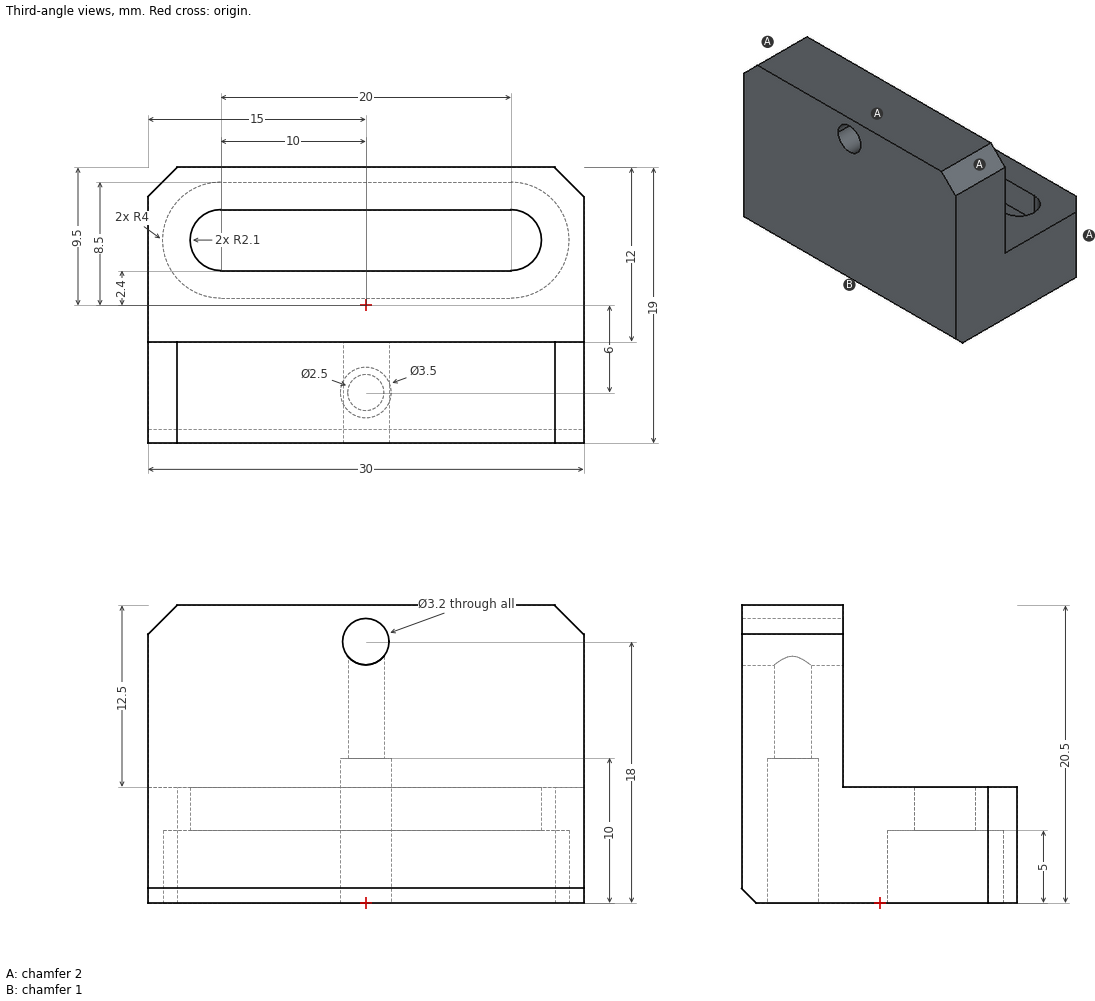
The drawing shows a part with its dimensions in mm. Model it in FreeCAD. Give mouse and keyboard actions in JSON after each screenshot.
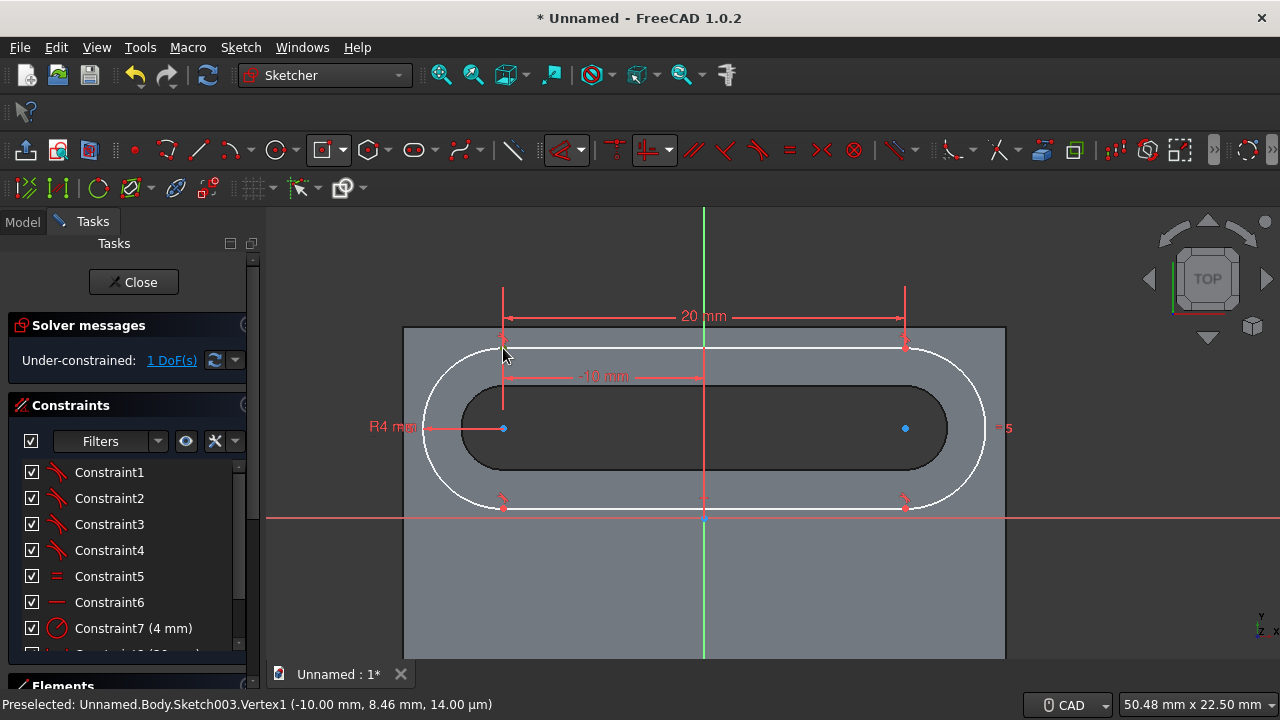
{"action": "left_click", "coordinate": [584, 150]}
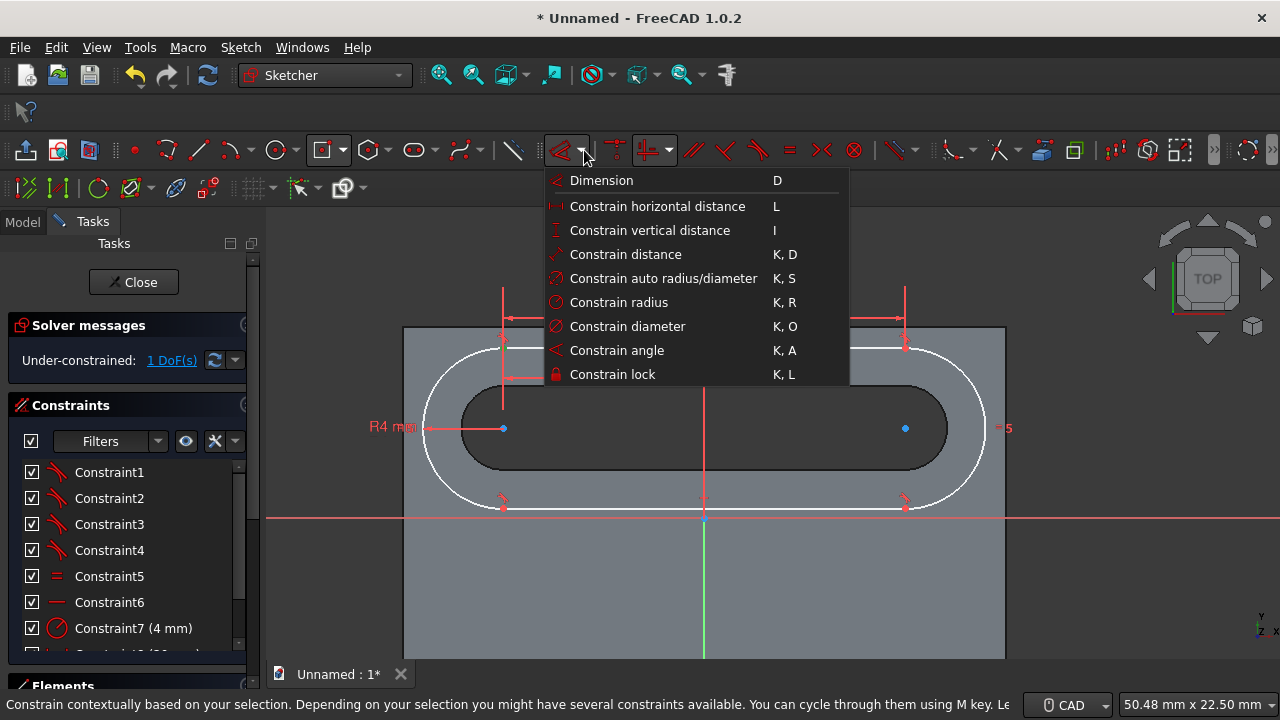
{"action": "left_click", "coordinate": [697, 230]}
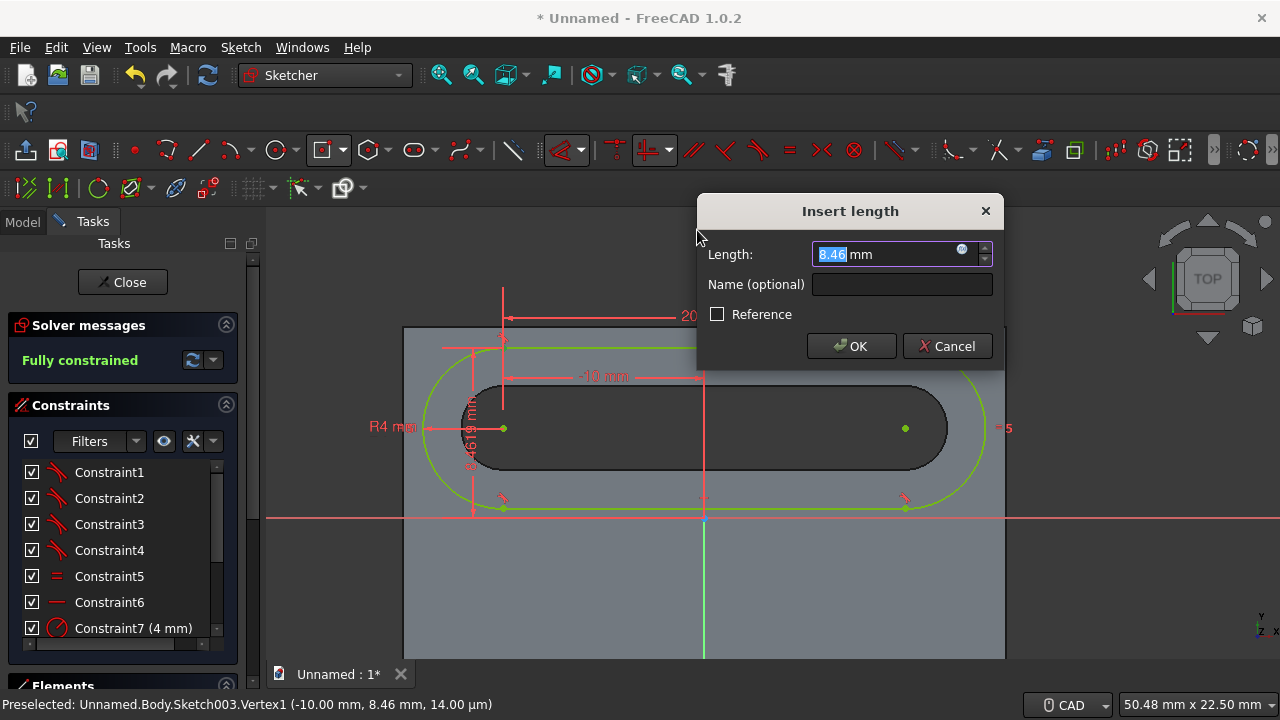
{"action": "type", "text": "8.5"}
{"action": "key", "text": "Return"}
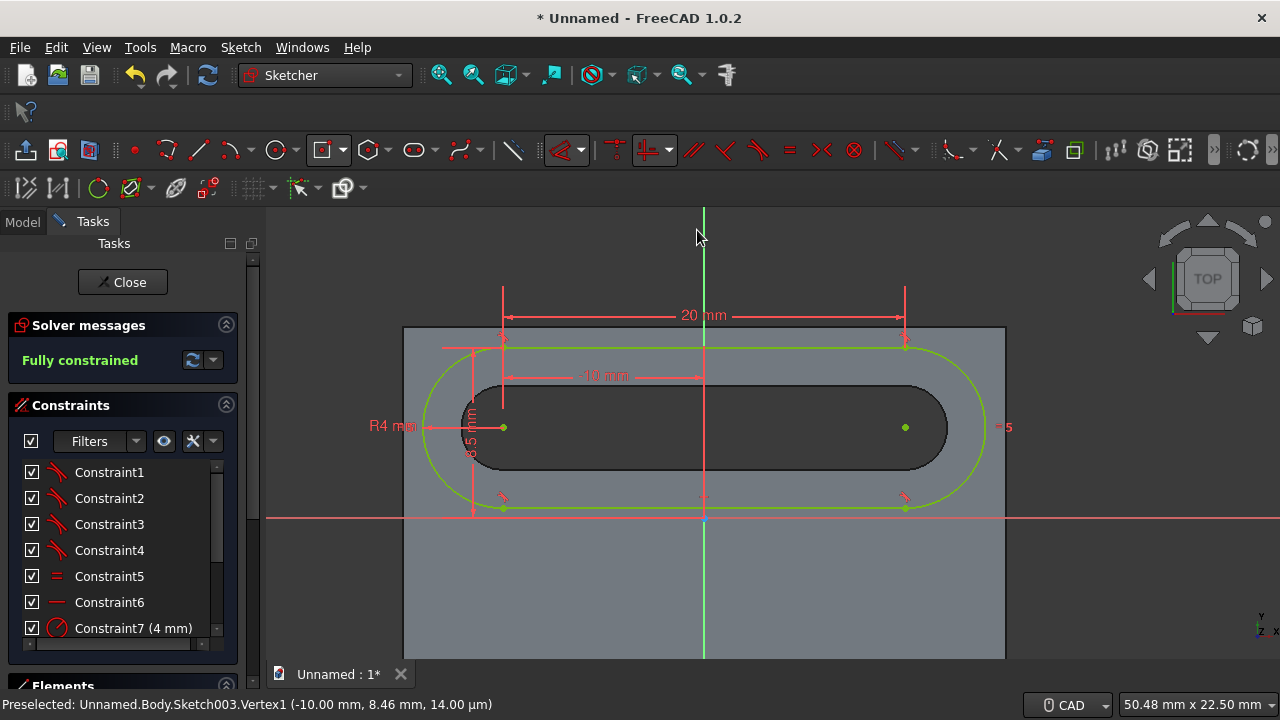
{"action": "left_click", "coordinate": [123, 282]}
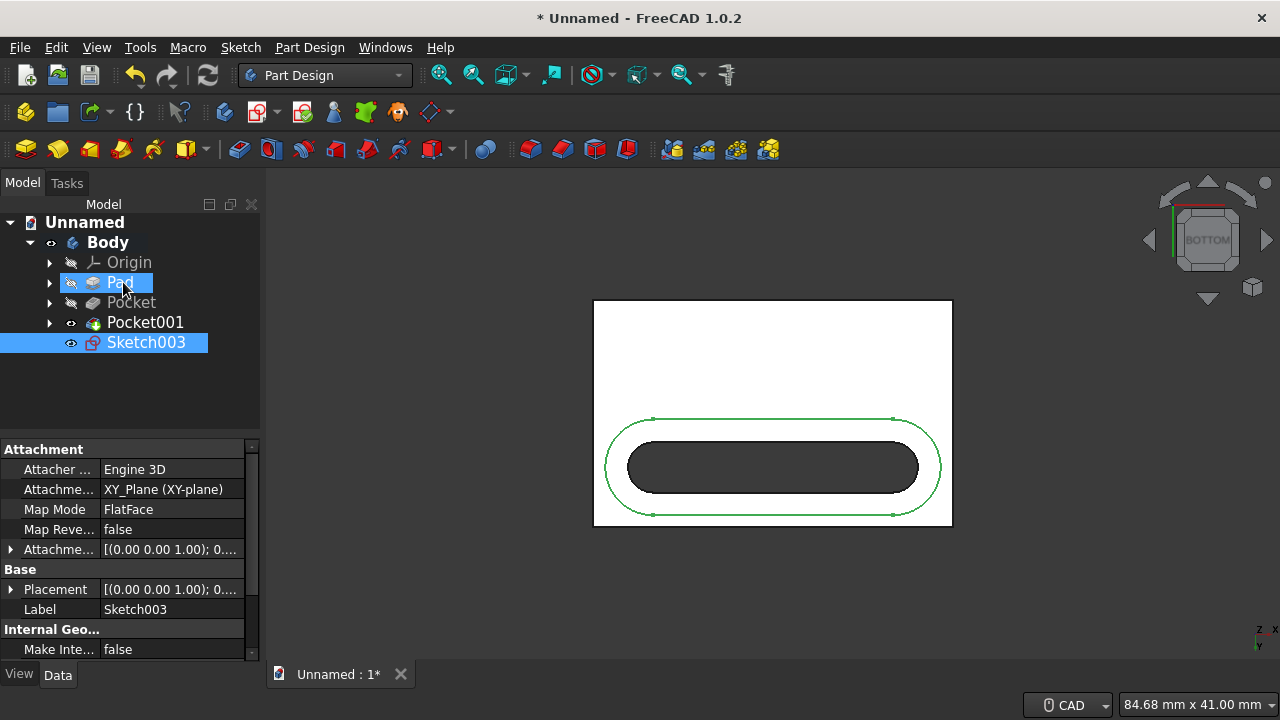
{"action": "left_click", "coordinate": [240, 150]}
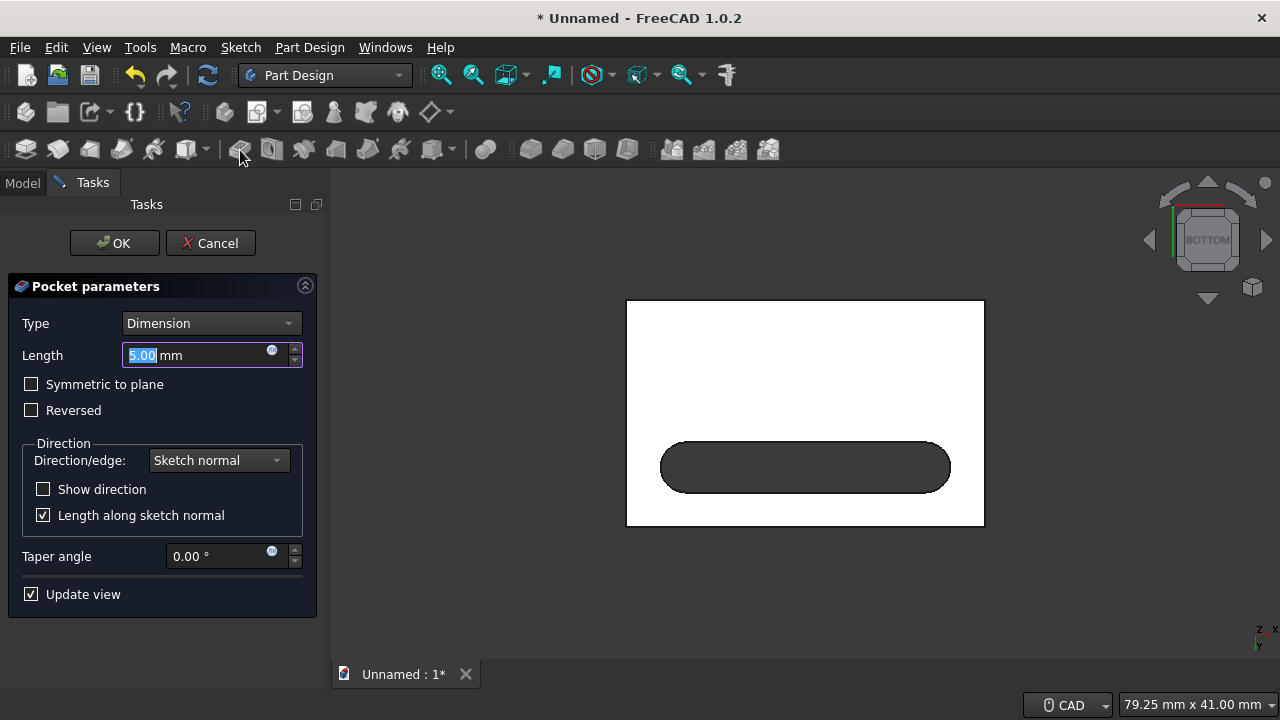
{"action": "type", "text": "5"}
{"action": "key", "text": "Tab"}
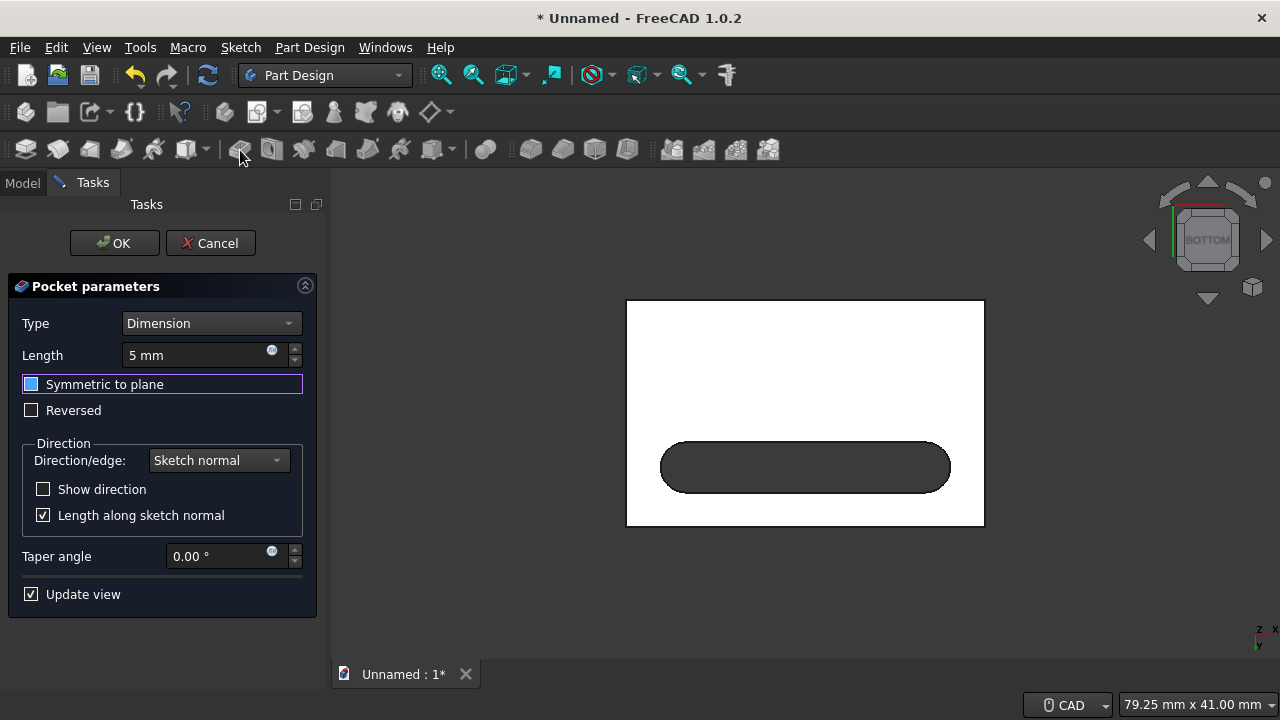
{"action": "left_click", "coordinate": [30, 410]}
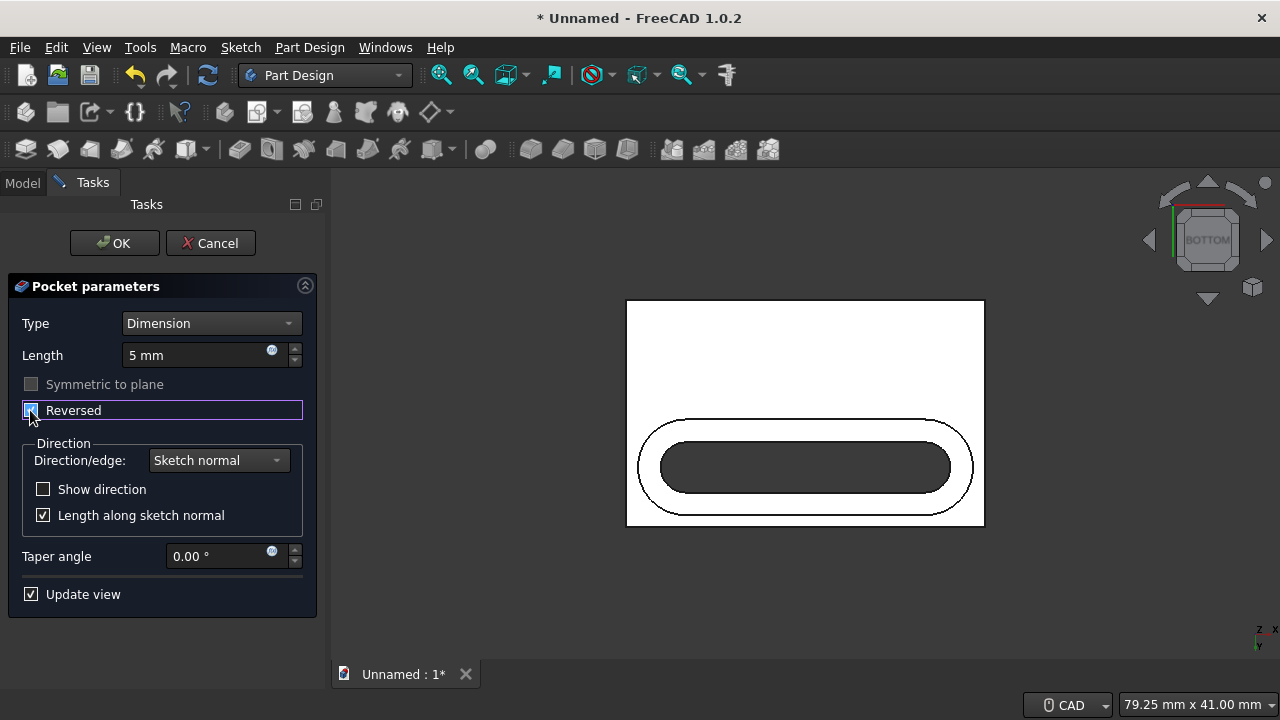
{"action": "left_click", "coordinate": [115, 243]}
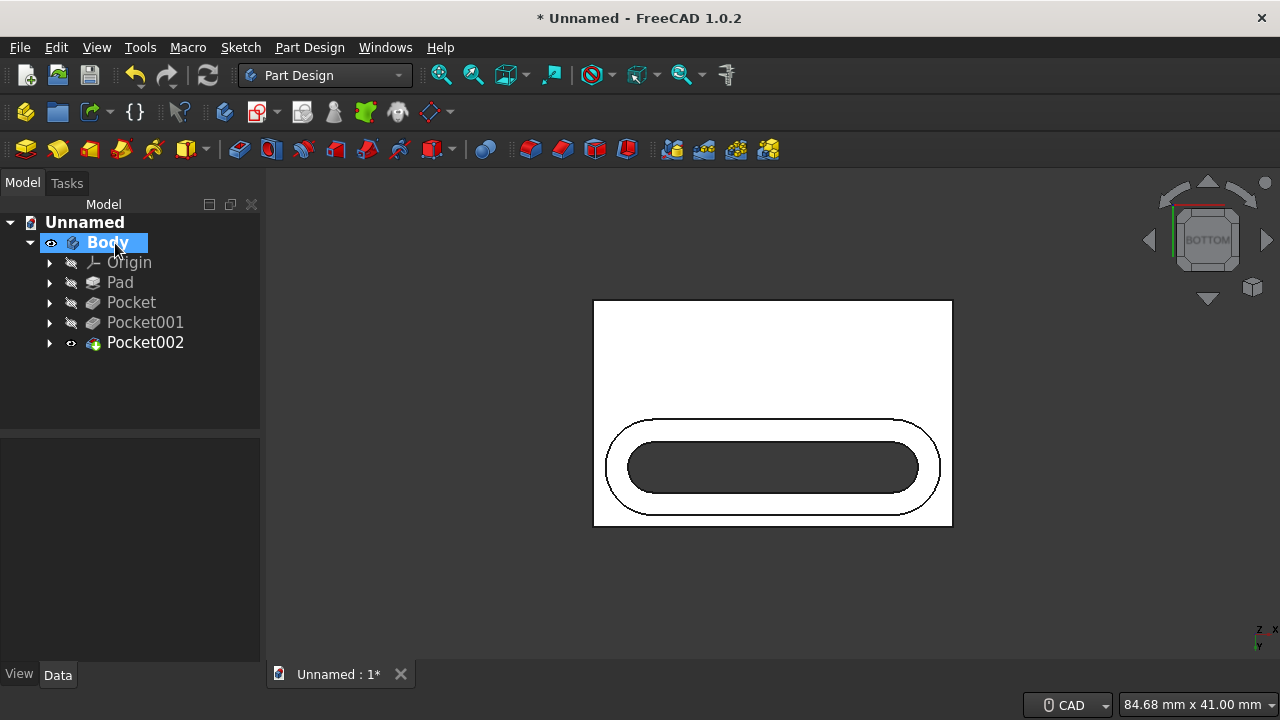
{"action": "left_click", "coordinate": [876, 347]}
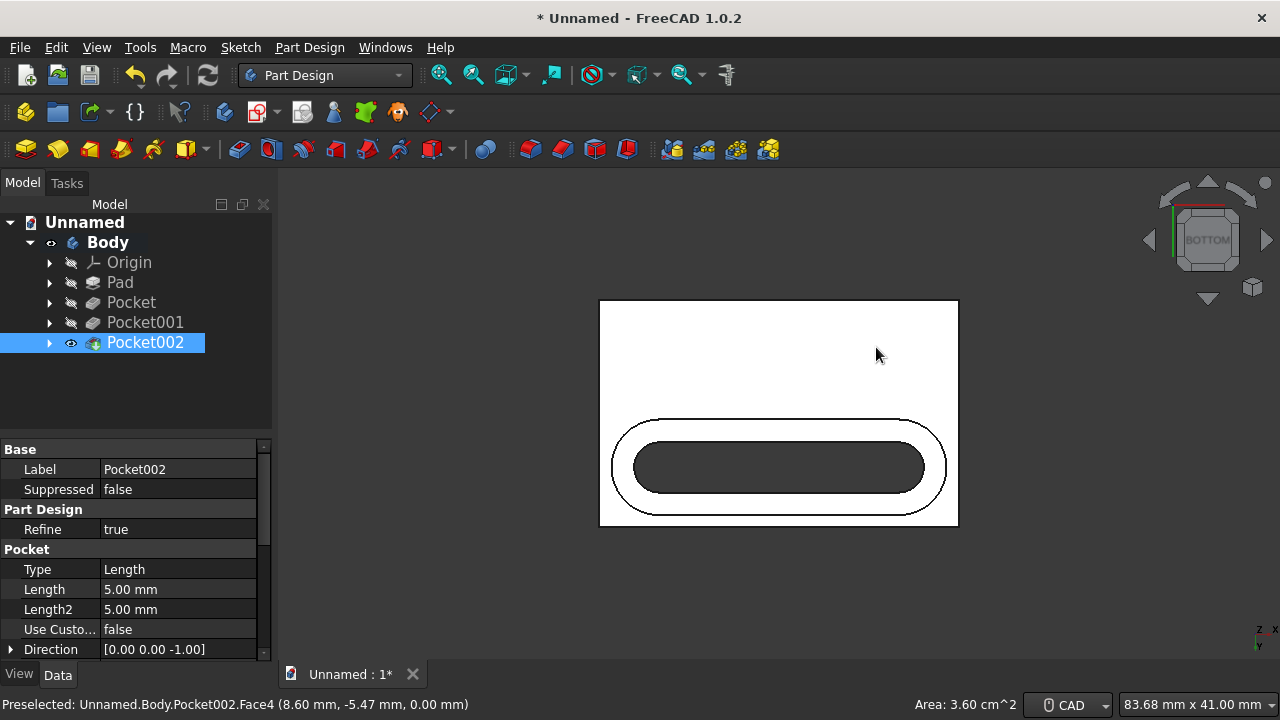
{"action": "left_click", "coordinate": [258, 112]}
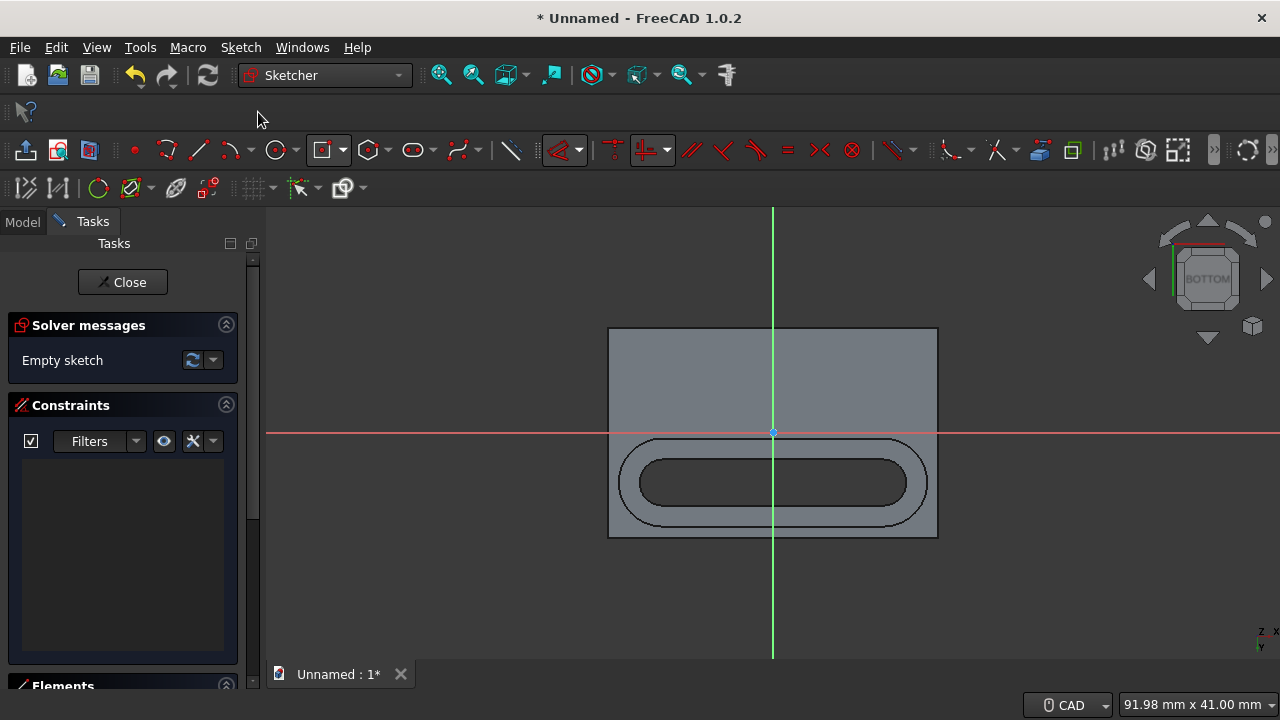
{"action": "scroll", "coordinate": [803, 372], "scroll_direction": "up", "scroll_amount": 6}